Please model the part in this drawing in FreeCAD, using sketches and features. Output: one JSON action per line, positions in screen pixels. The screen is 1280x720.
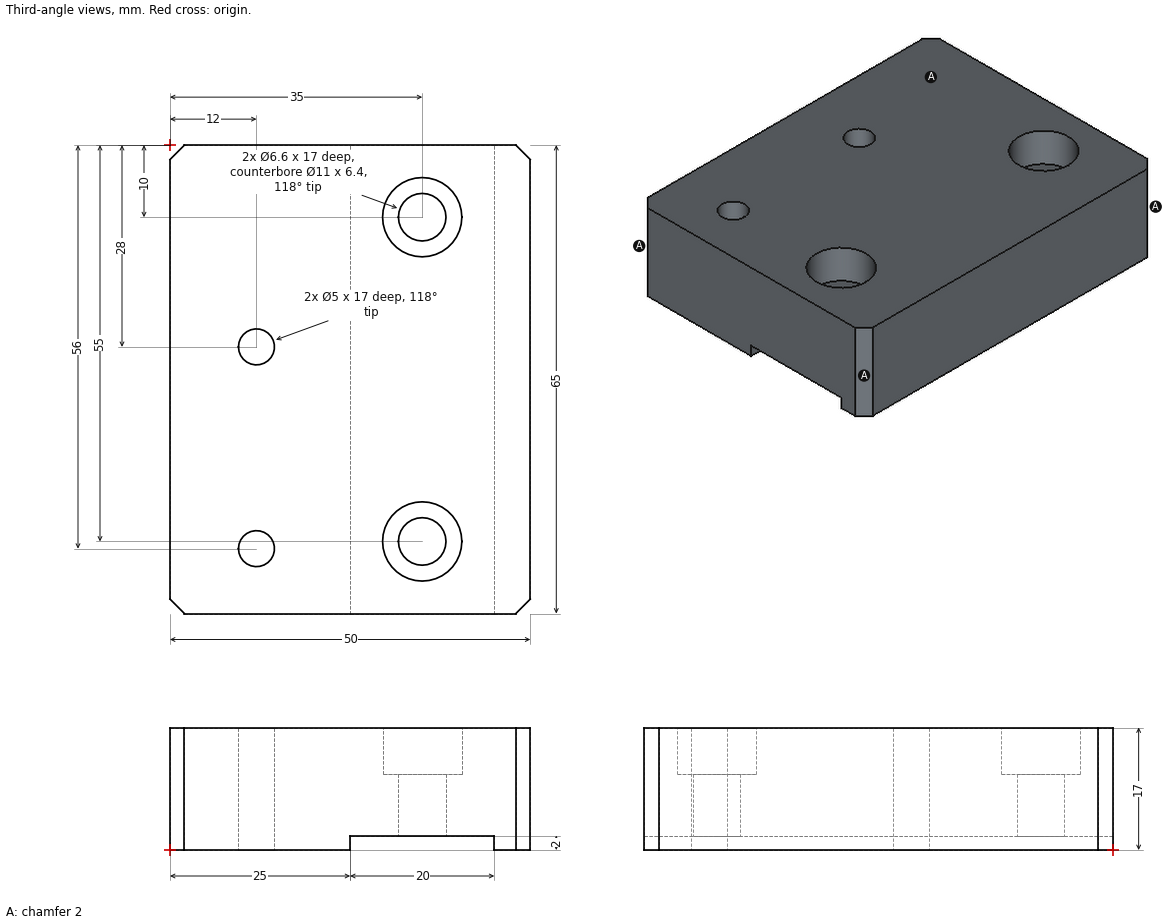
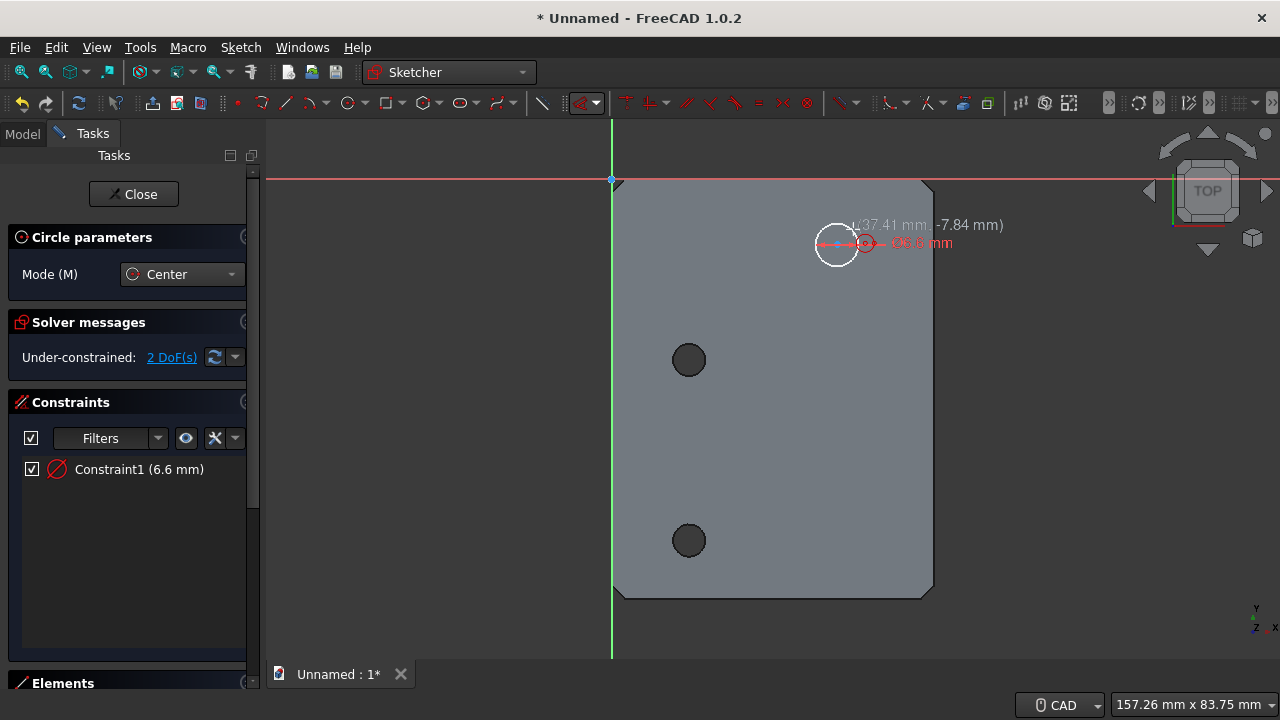
{"action": "left_click", "coordinate": [837, 534]}
{"action": "mouse_move", "coordinate": [853, 519]}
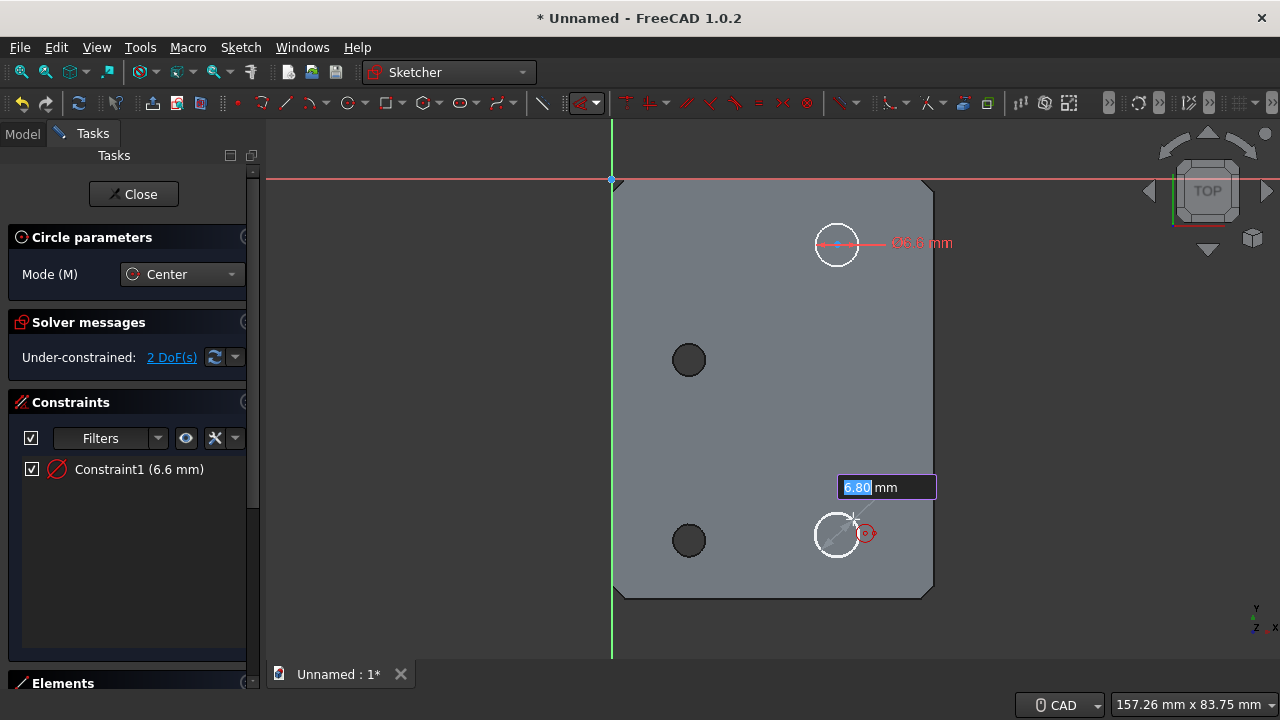
{"action": "type", "text": "6.6"}
{"action": "key", "text": "Return"}
{"action": "key", "text": "Escape"}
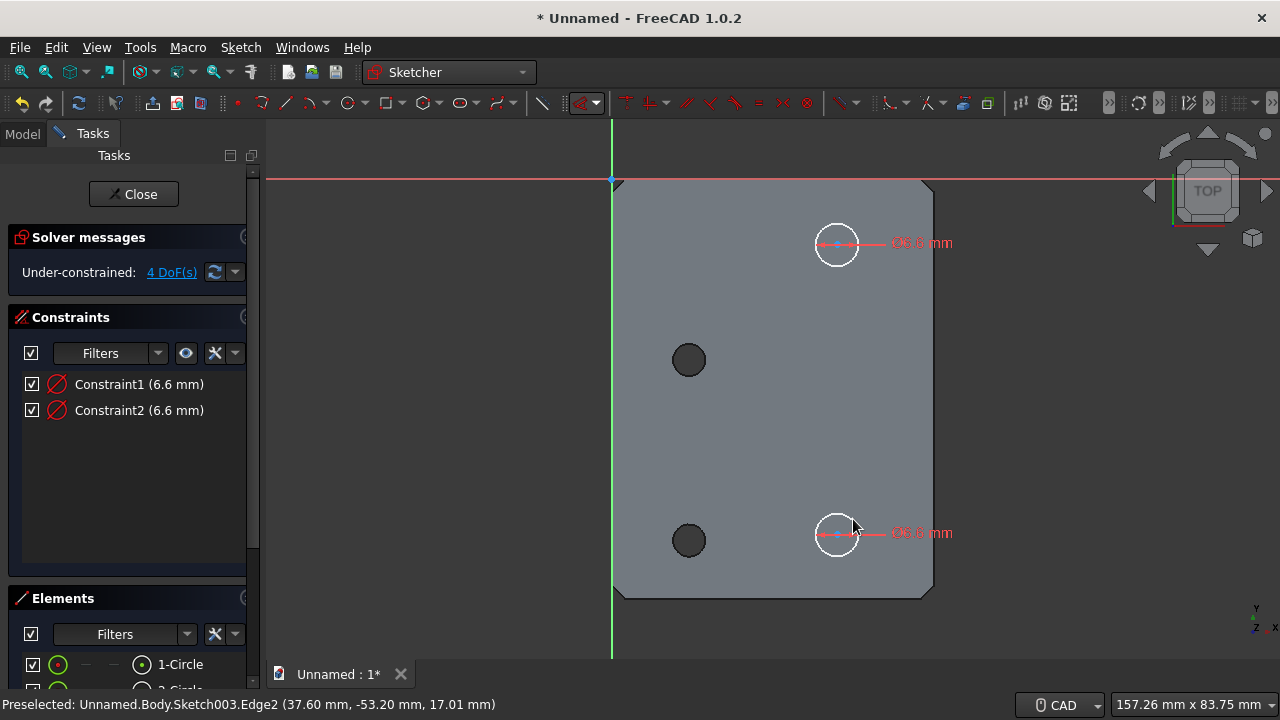
{"action": "left_click", "coordinate": [837, 245]}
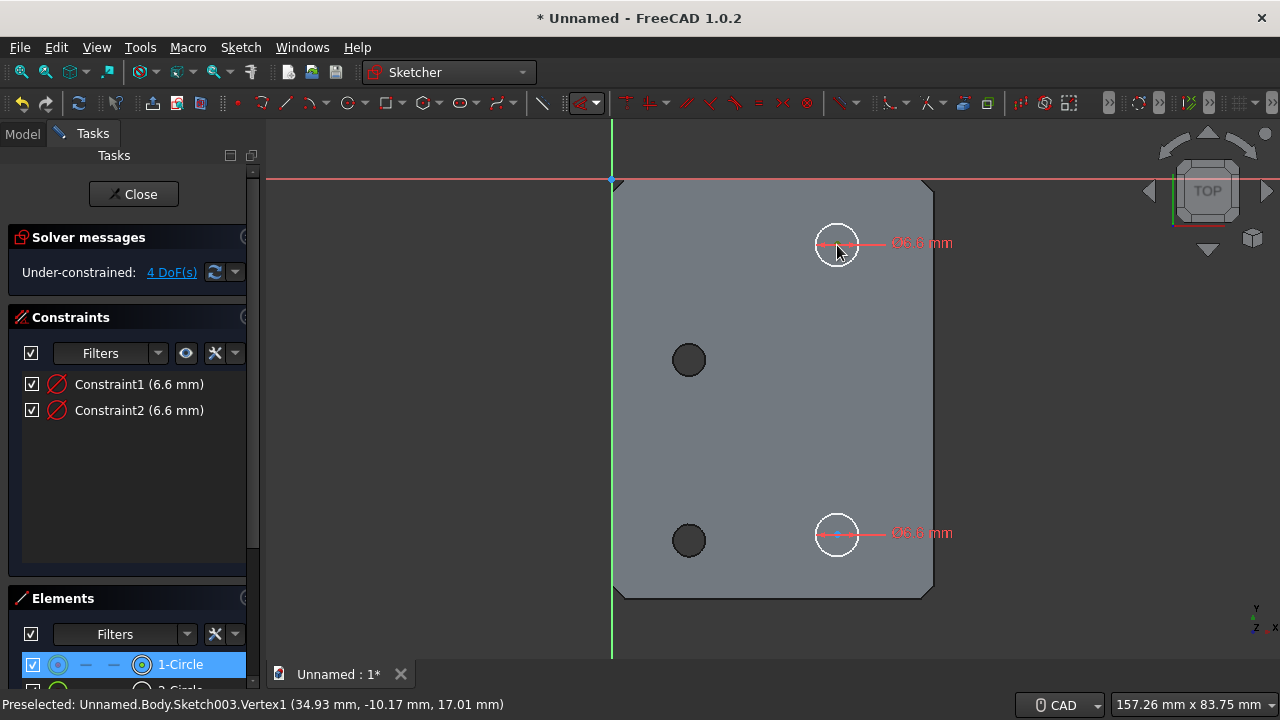
{"action": "key", "text": "l"}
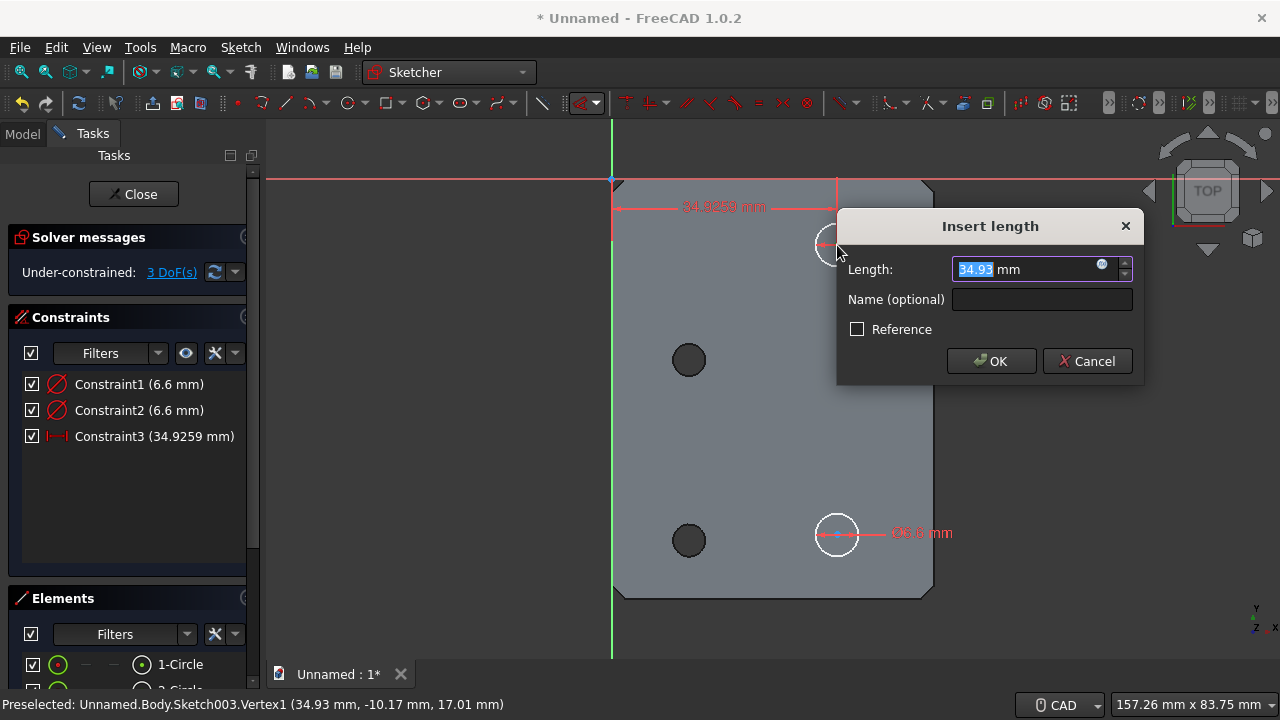
{"action": "type", "text": "35"}
{"action": "key", "text": "Return"}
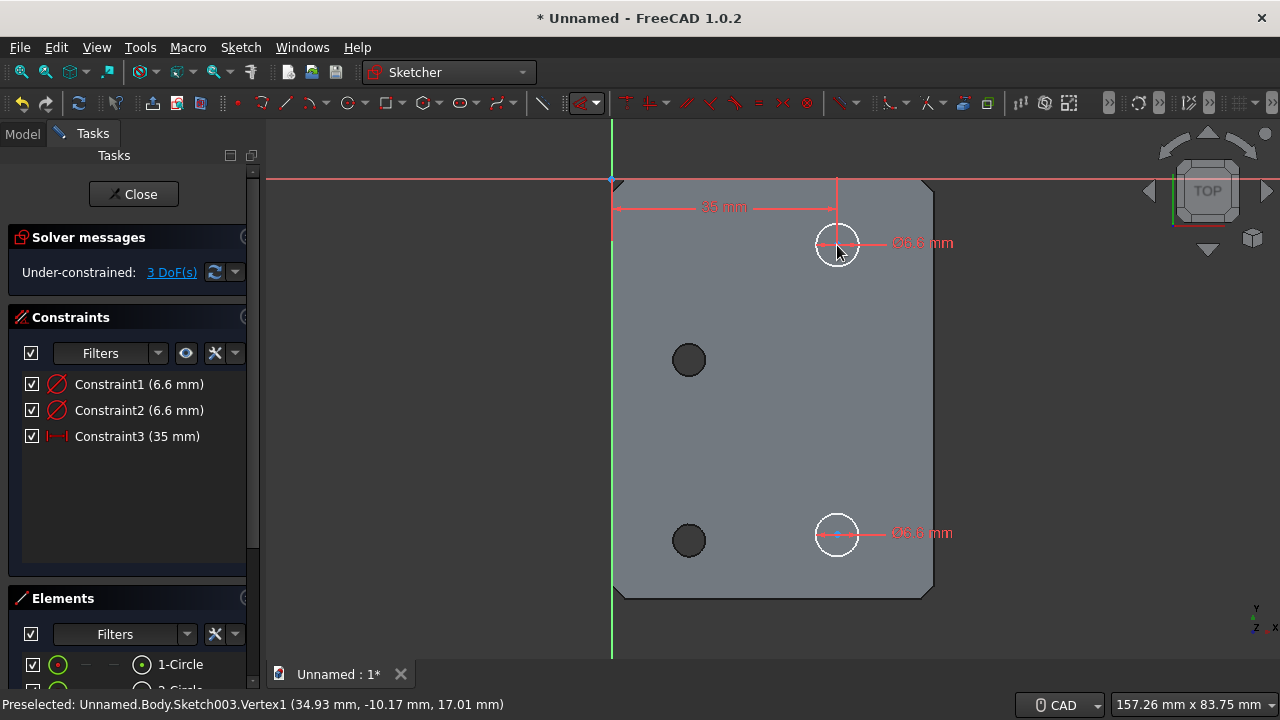
{"action": "left_click", "coordinate": [837, 245]}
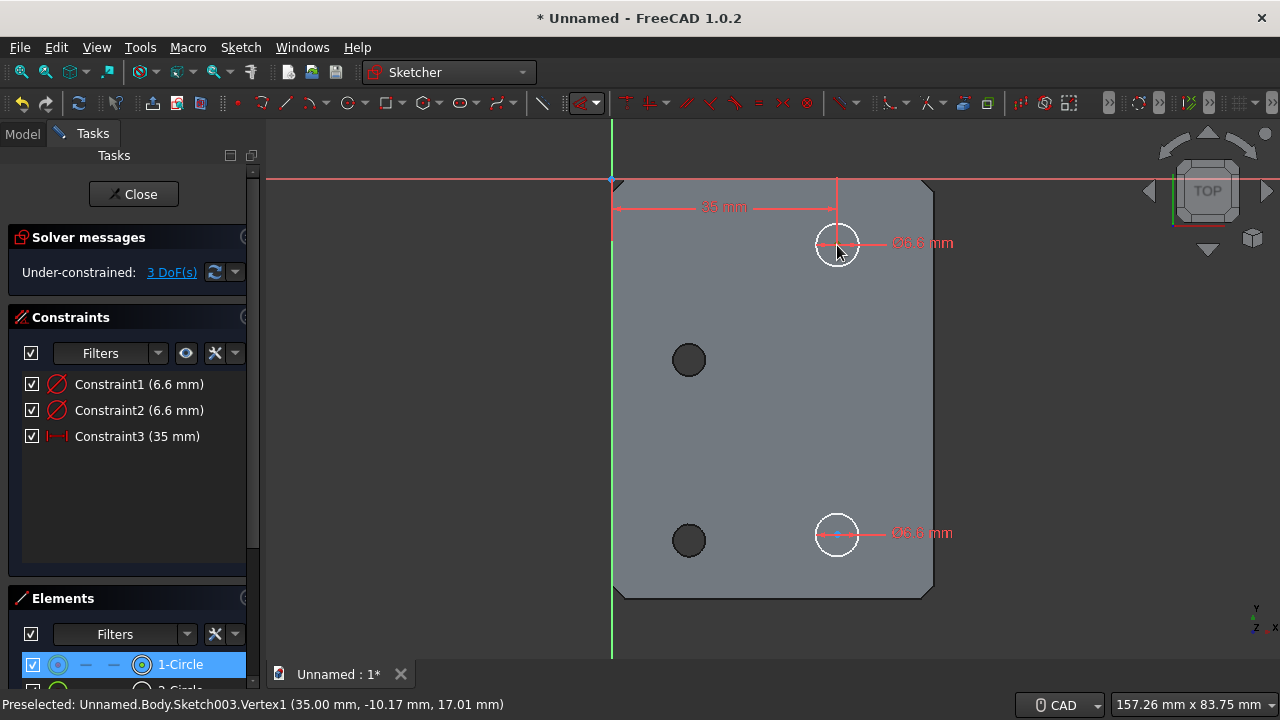
{"action": "left_click", "coordinate": [598, 104]}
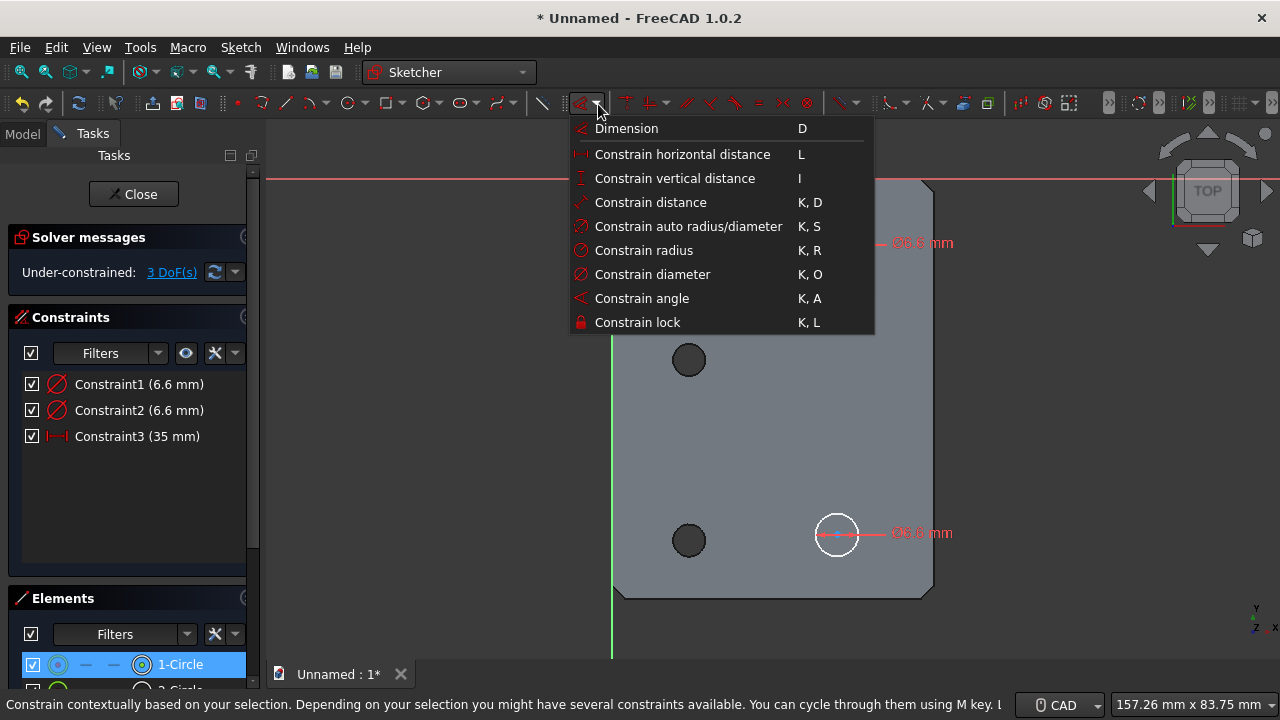
{"action": "left_click", "coordinate": [722, 178]}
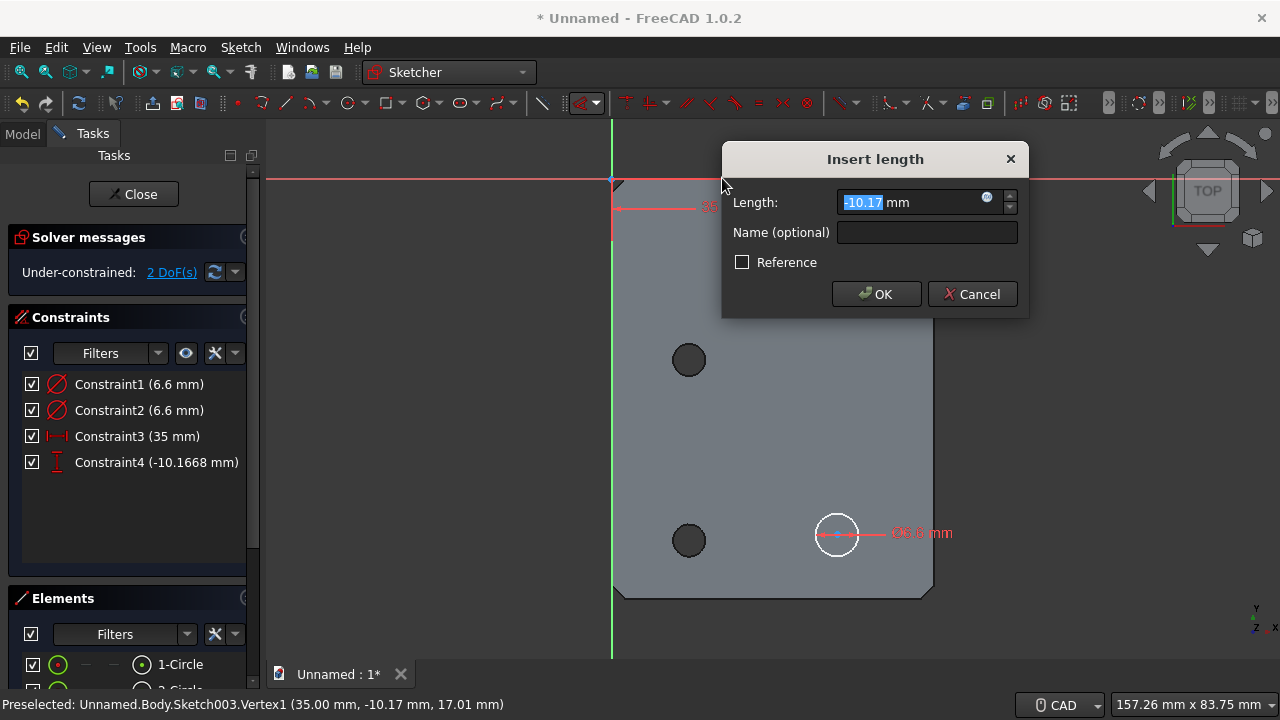
{"action": "type", "text": "-10"}
{"action": "key", "text": "Return"}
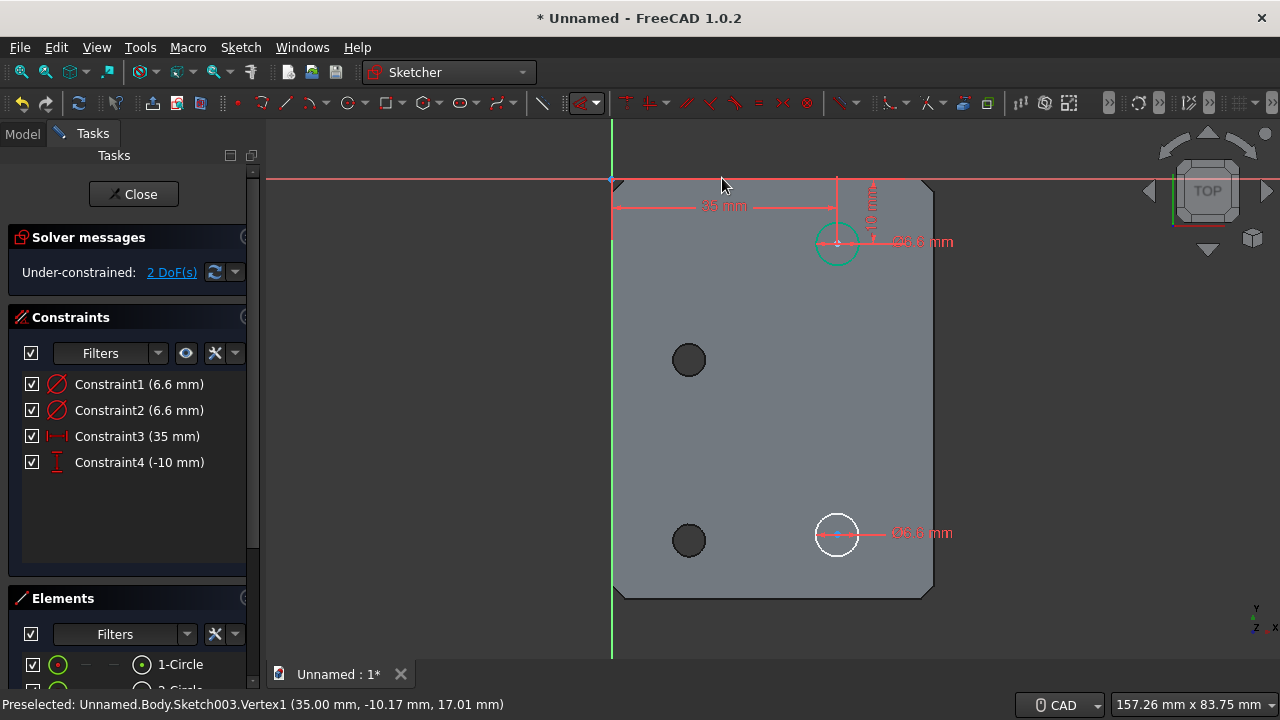
{"action": "left_click", "coordinate": [837, 535]}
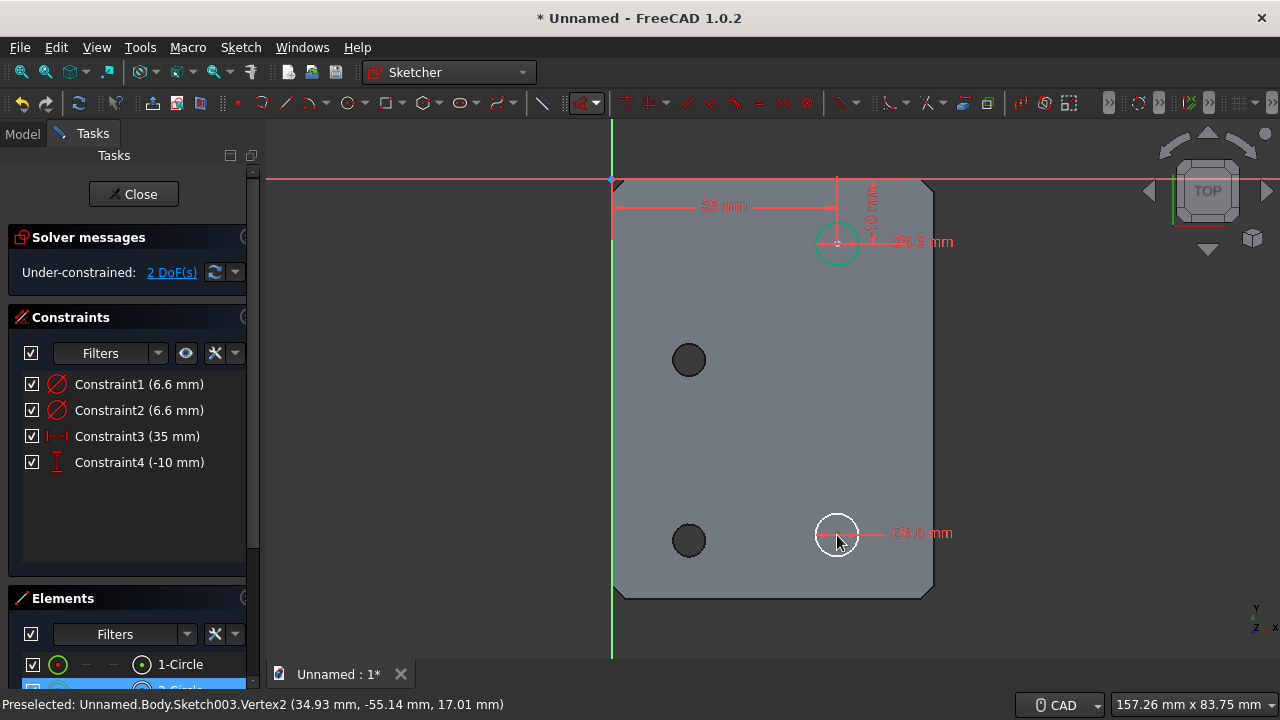
{"action": "key", "text": "l"}